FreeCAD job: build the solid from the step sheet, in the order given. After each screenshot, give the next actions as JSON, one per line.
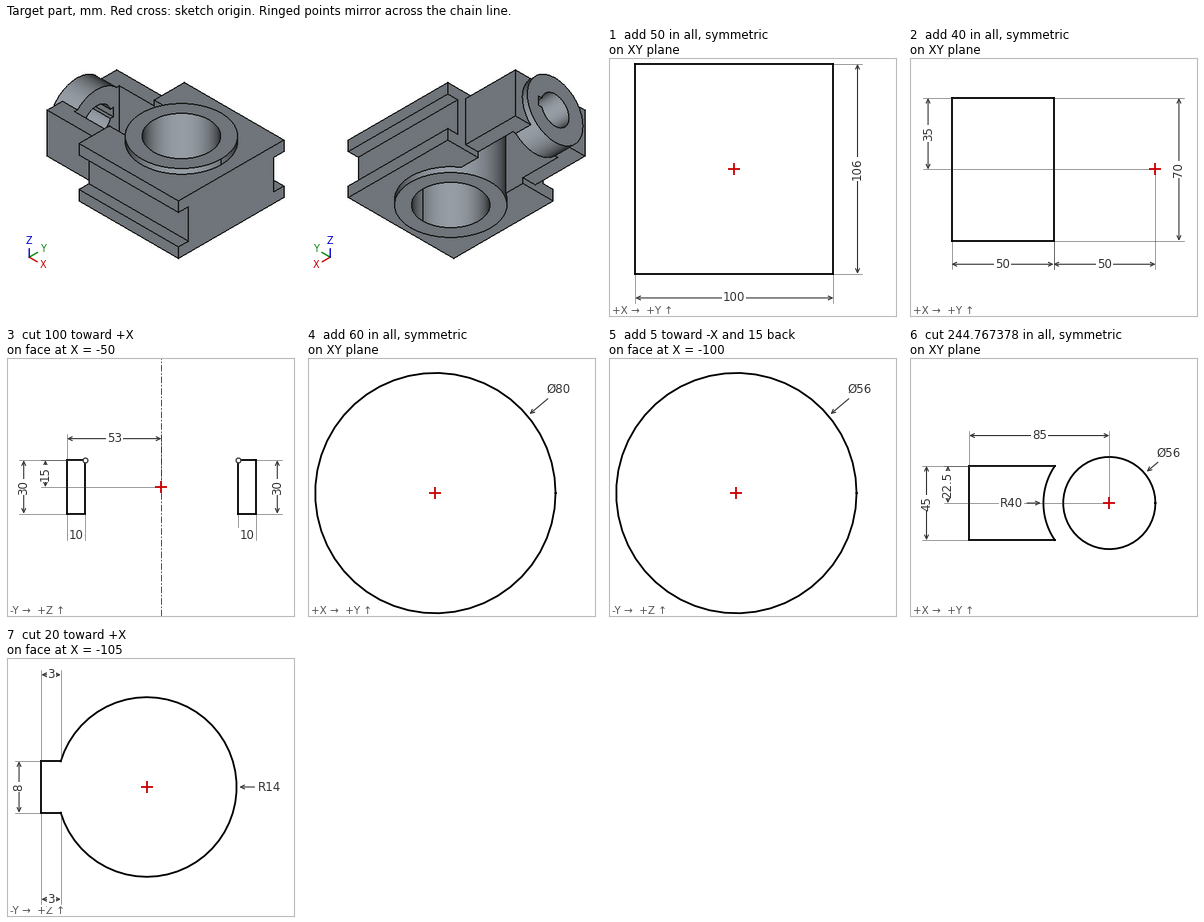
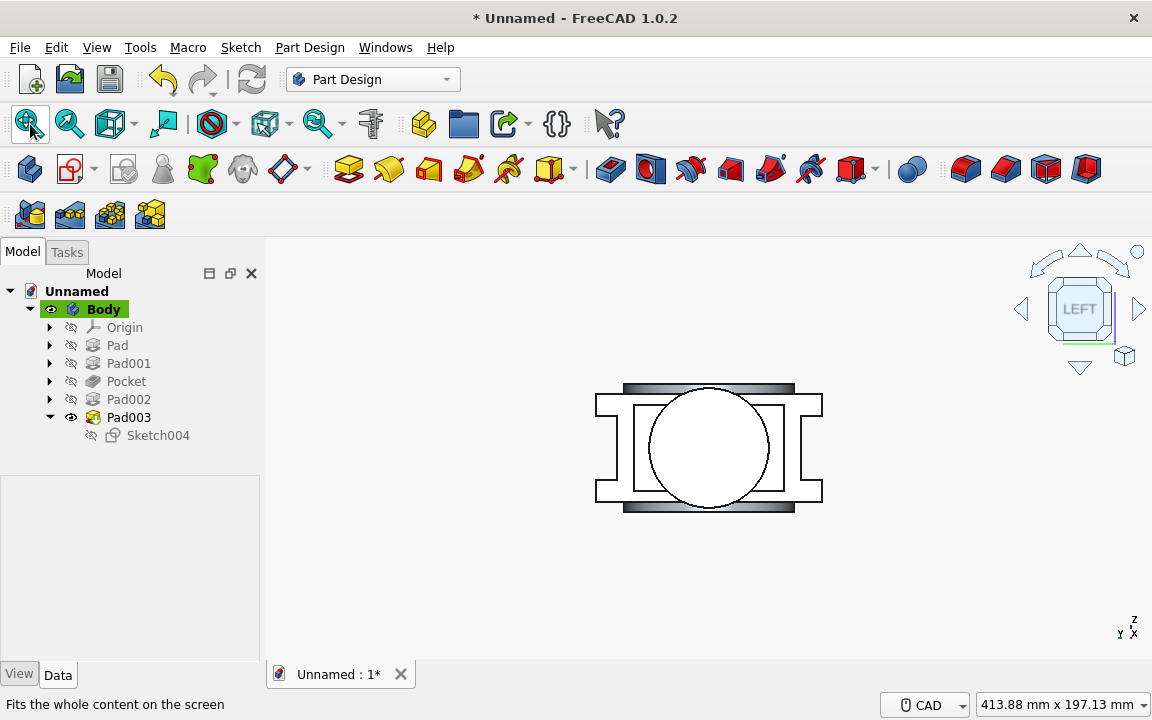
{"action": "left_click", "coordinate": [70, 170]}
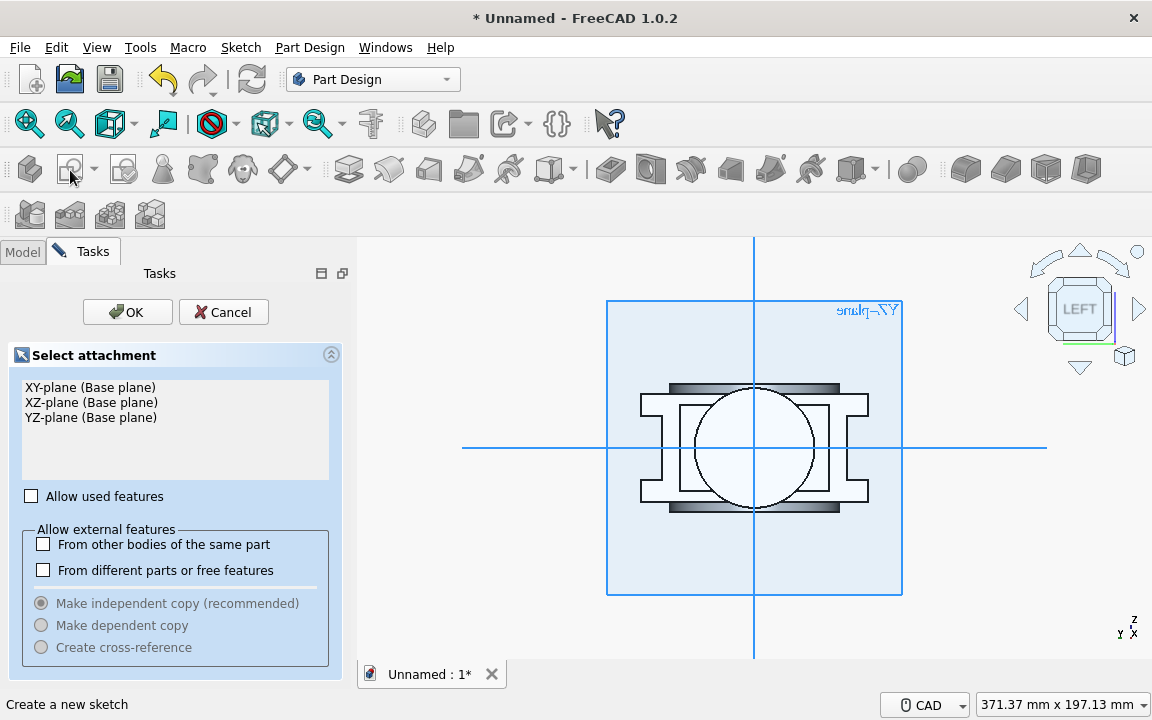
{"action": "left_click", "coordinate": [82, 388]}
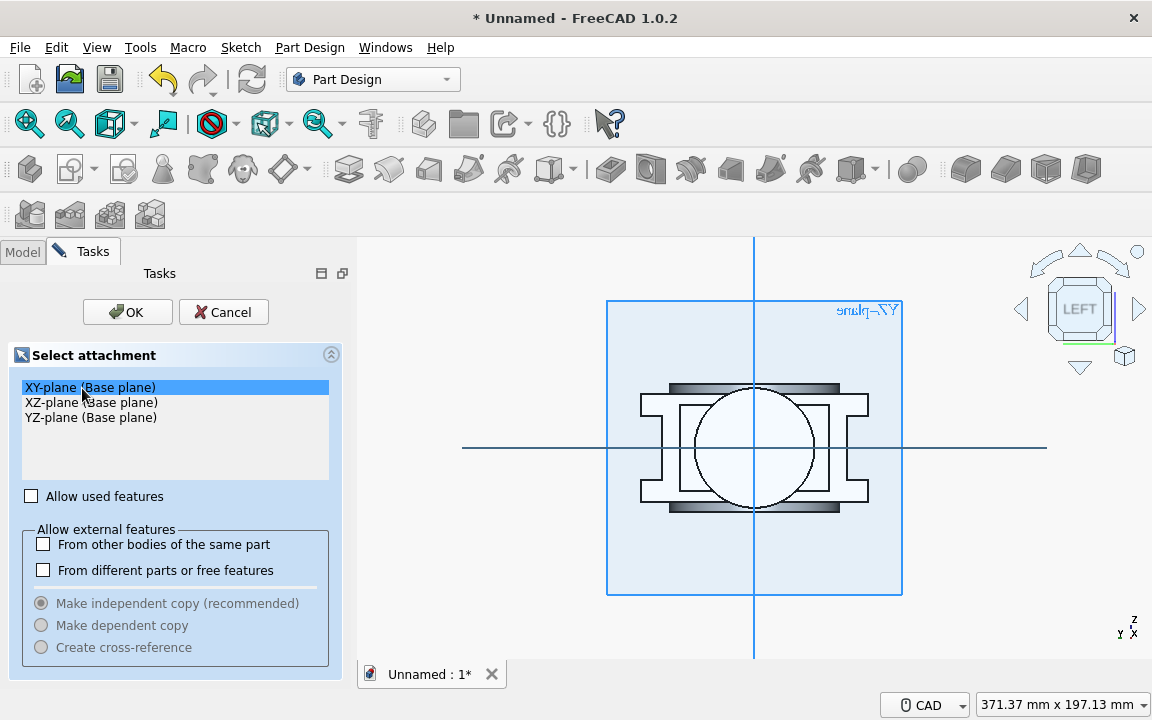
{"action": "left_click", "coordinate": [128, 312]}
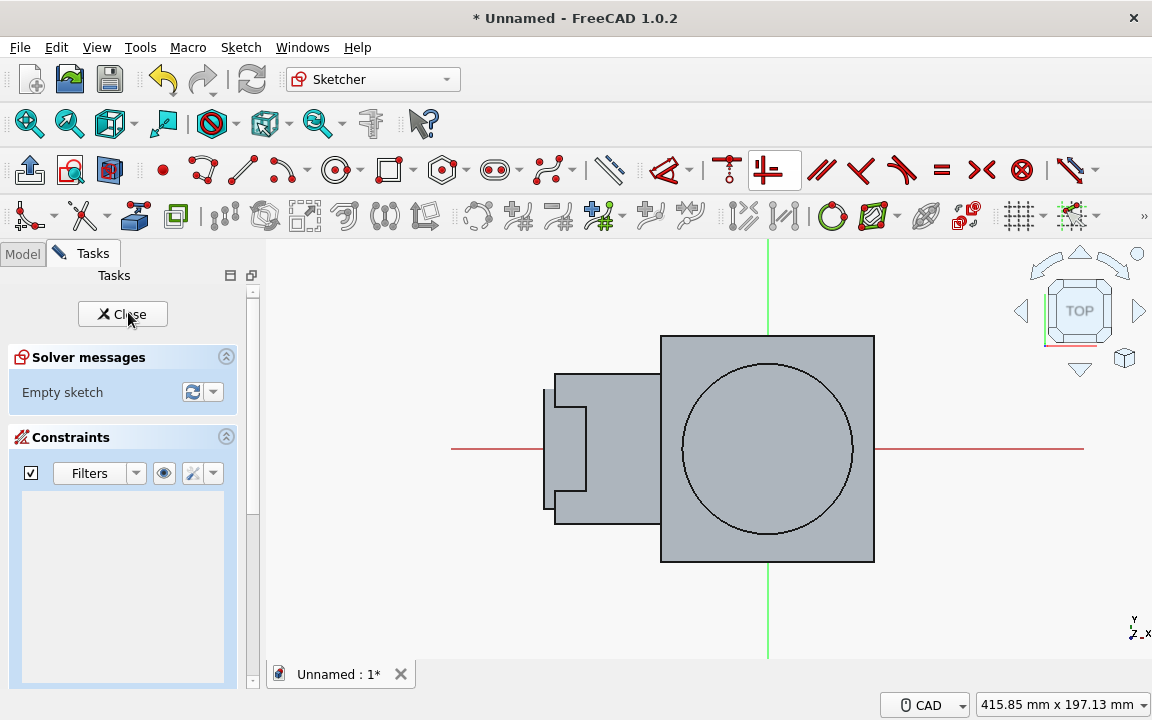
{"action": "left_click", "coordinate": [110, 170]}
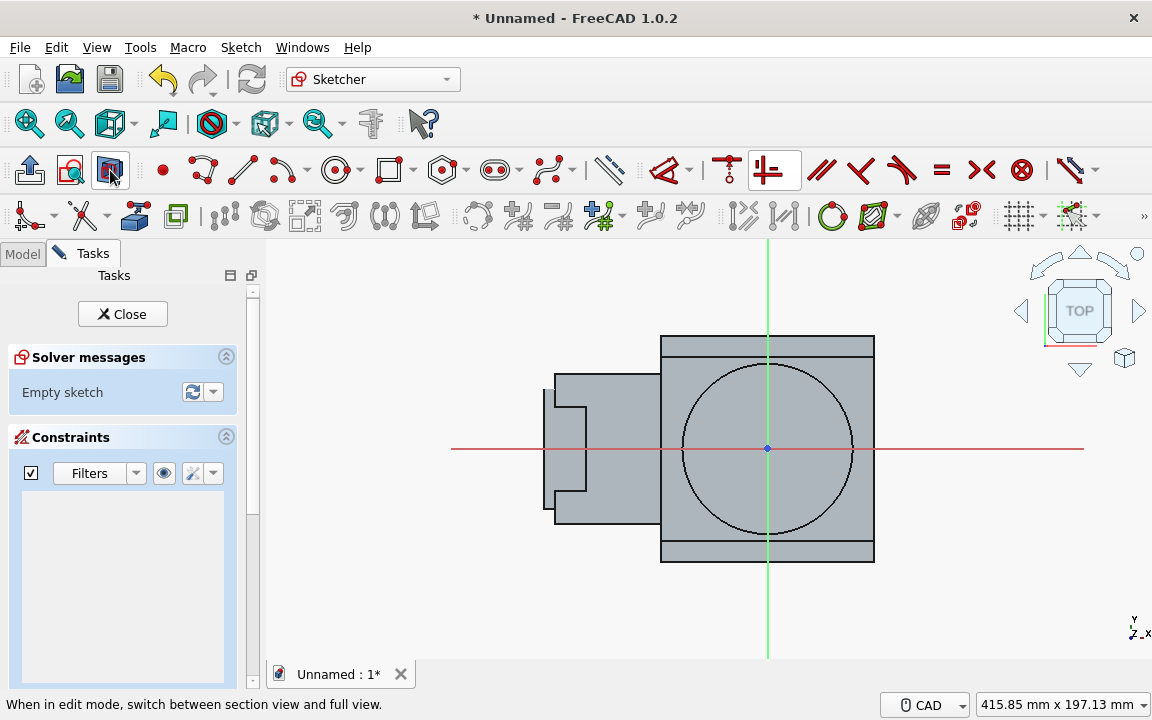
{"action": "scroll", "coordinate": [761, 449], "scroll_direction": "up", "scroll_amount": 4}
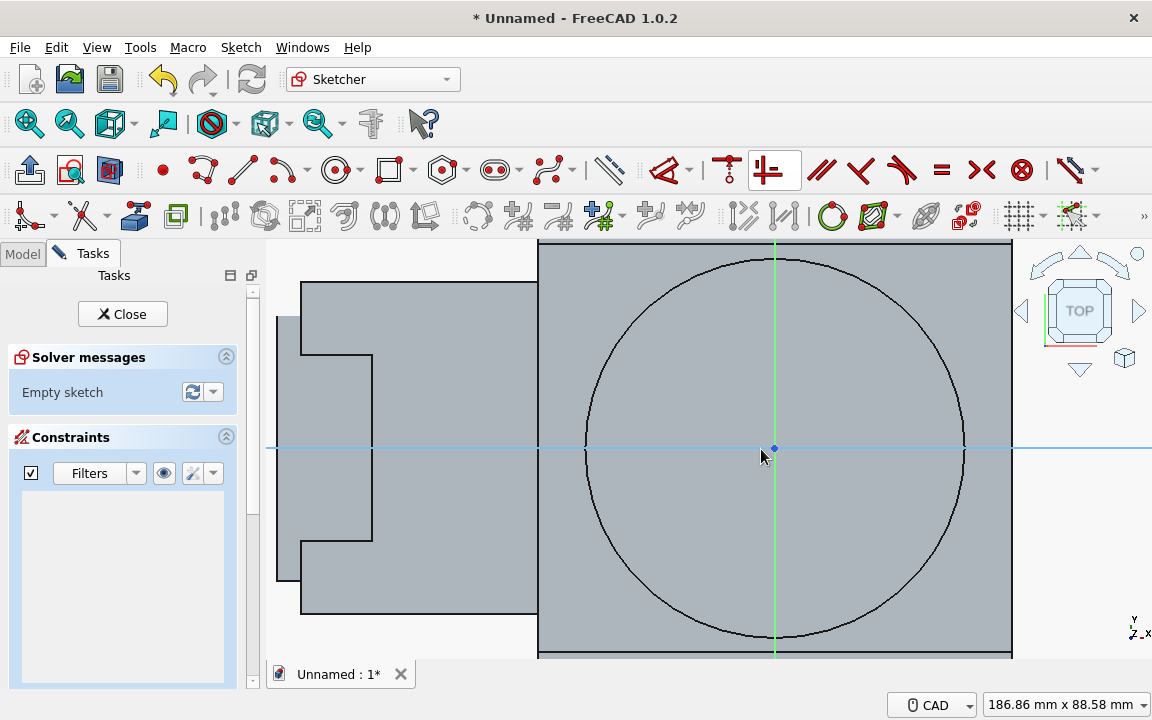
{"action": "left_click", "coordinate": [204, 170]}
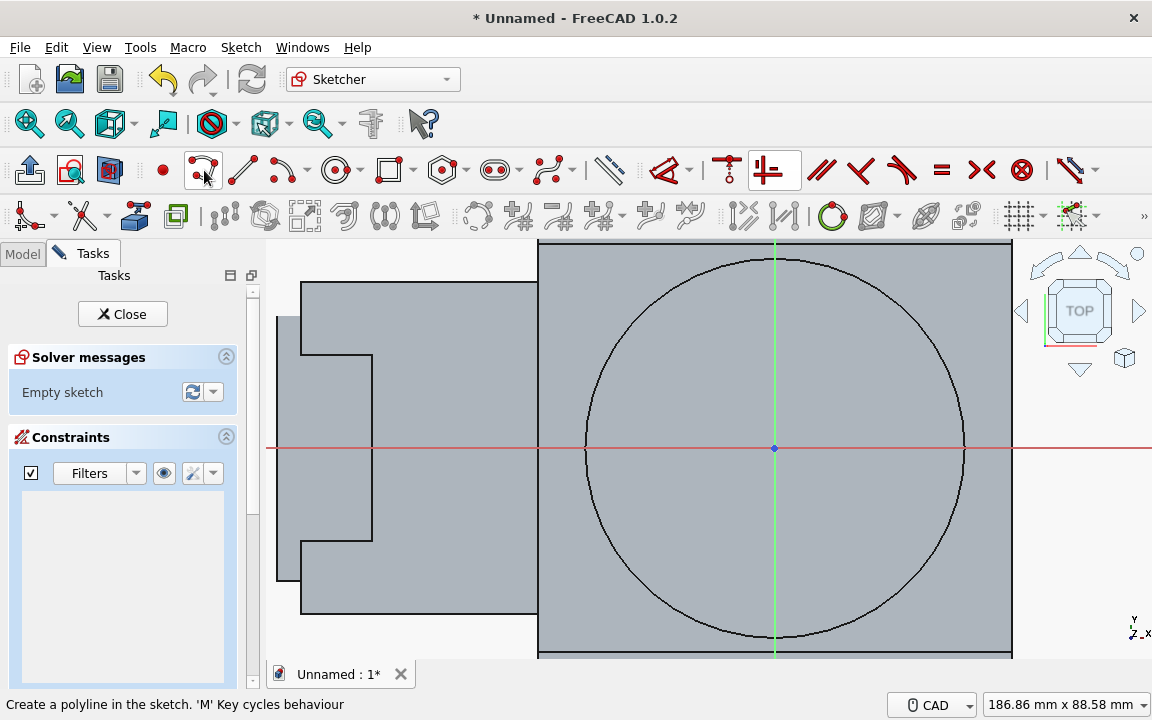
{"action": "left_click", "coordinate": [618, 342]}
{"action": "left_click", "coordinate": [372, 342]}
{"action": "left_click", "coordinate": [372, 555]}
{"action": "left_click", "coordinate": [618, 555]}
{"action": "right_click", "coordinate": [618, 555]}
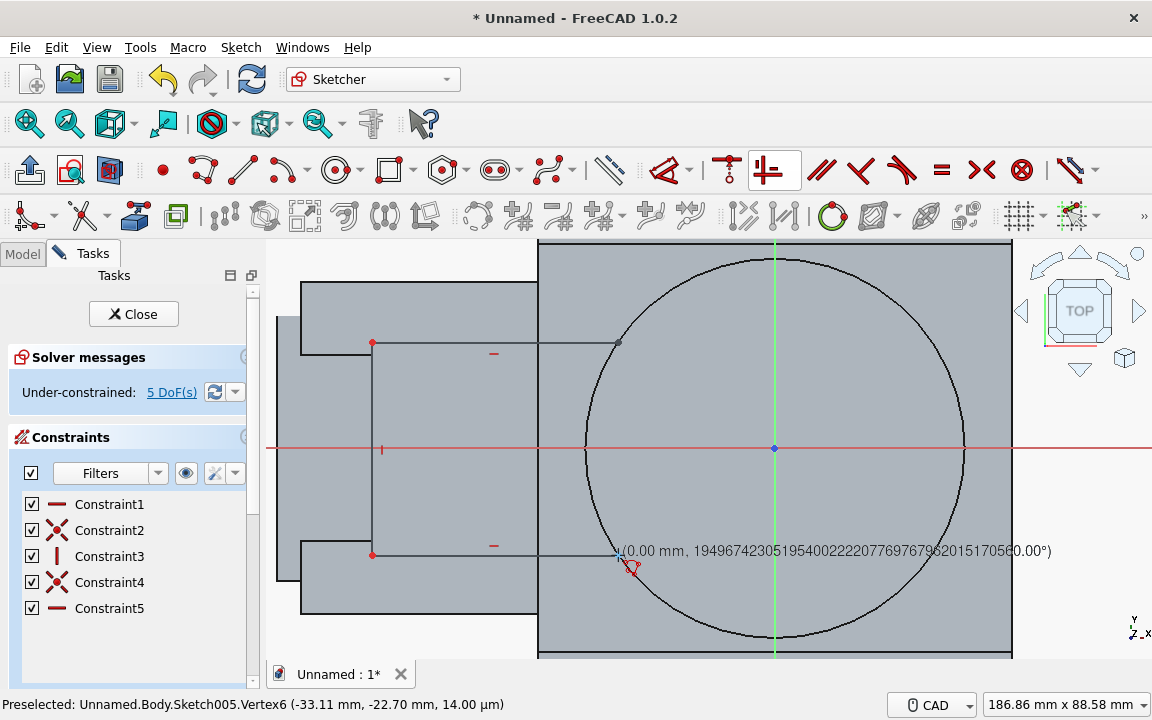
{"action": "key", "text": "g 3 a"}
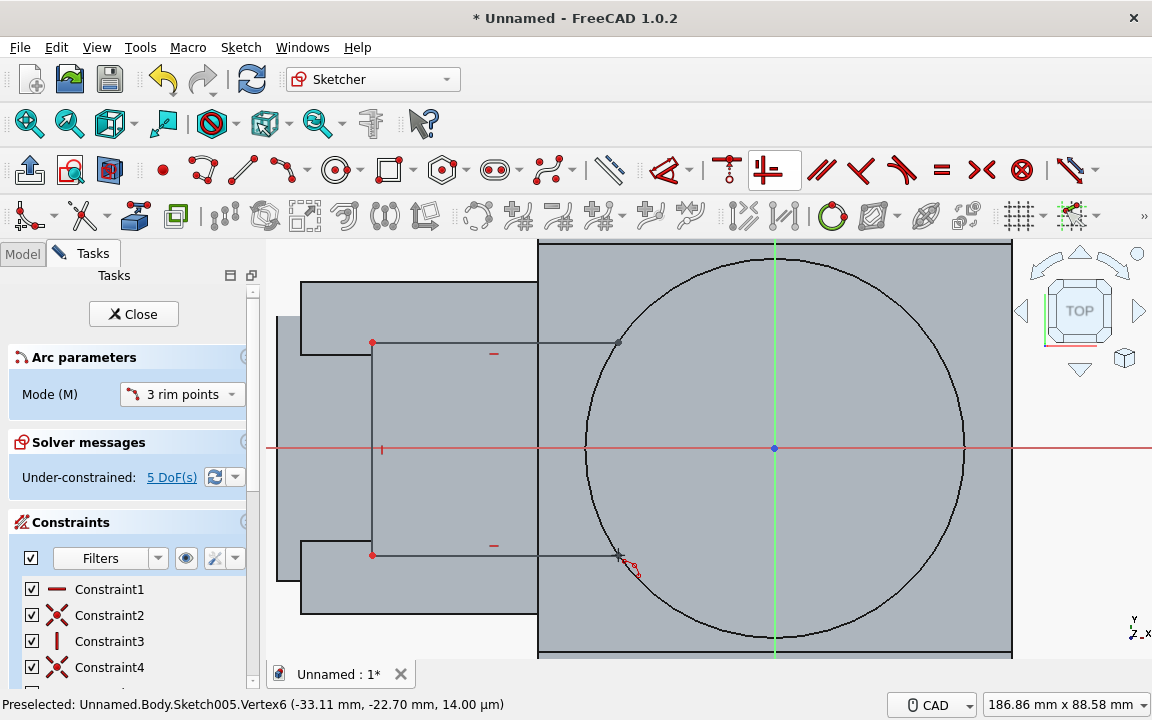
{"action": "left_click", "coordinate": [618, 556]}
{"action": "left_click", "coordinate": [618, 343]}
{"action": "left_click", "coordinate": [587, 426]}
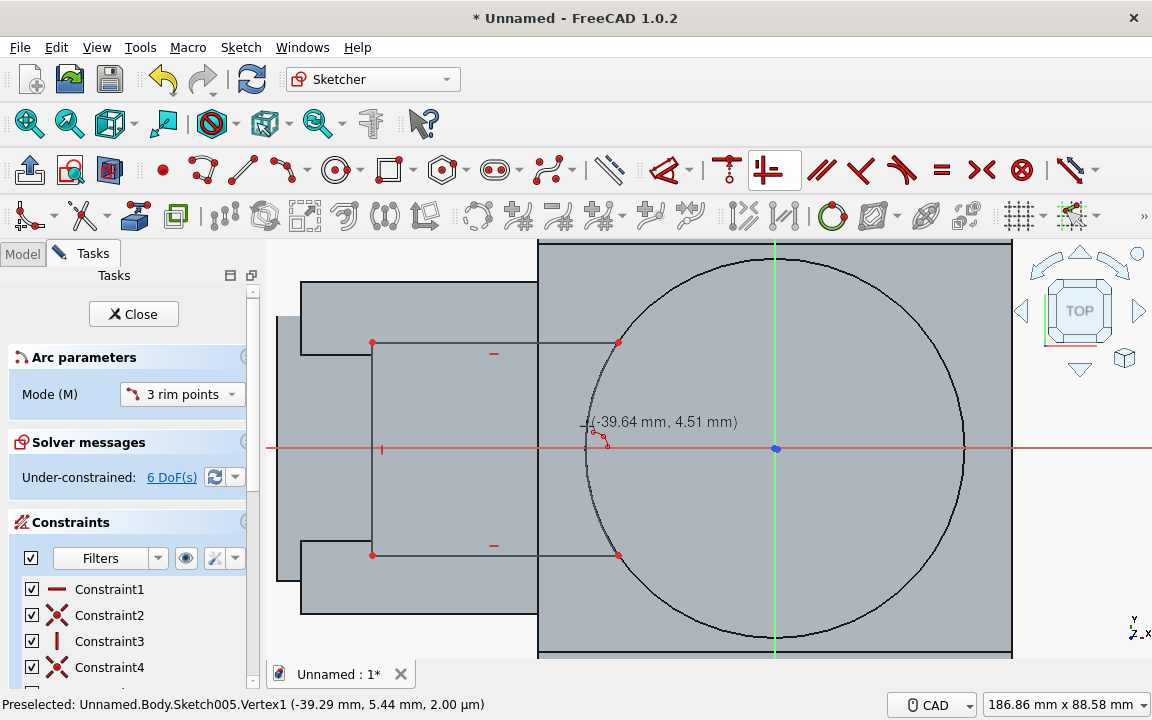
{"action": "left_click", "coordinate": [336, 170]}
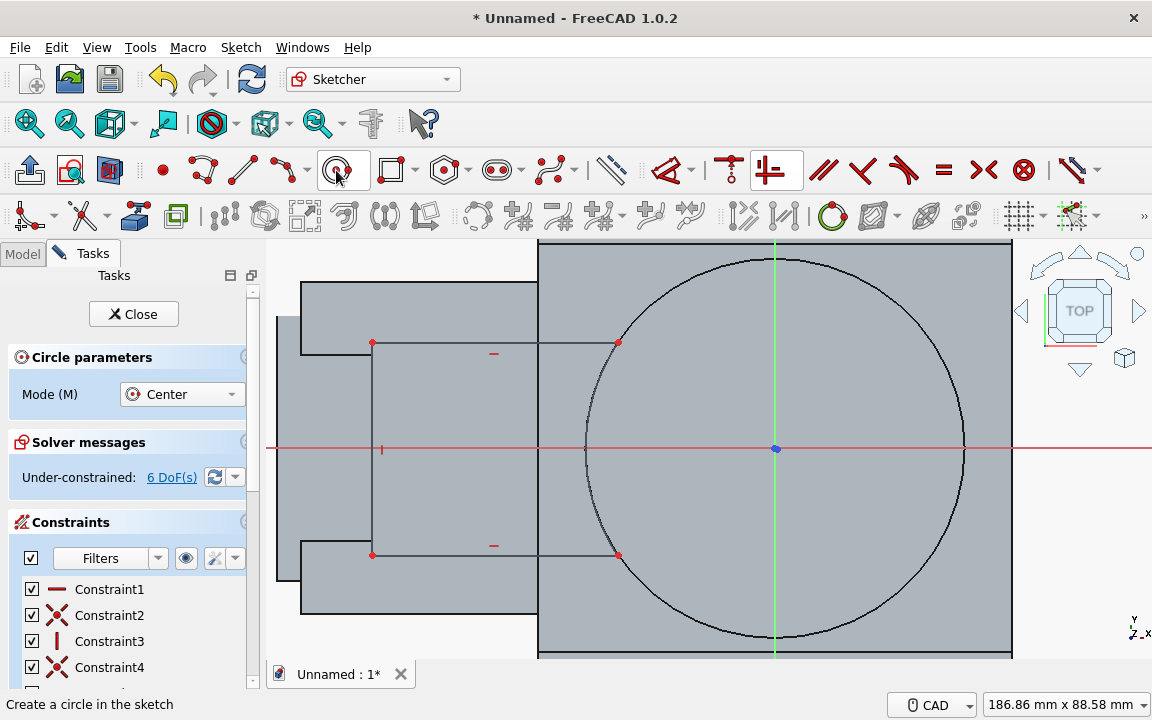
{"action": "left_click", "coordinate": [775, 448]}
{"action": "mouse_move", "coordinate": [869, 355]}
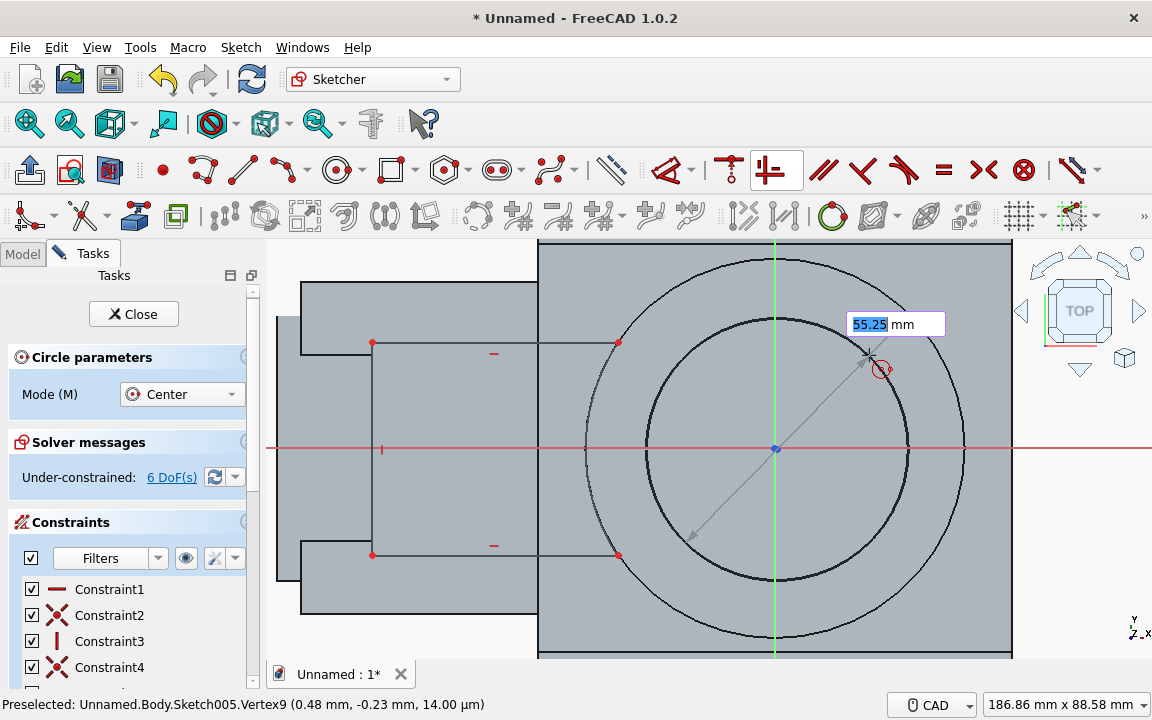
{"action": "type", "text": "56"}
{"action": "key", "text": "Return"}
{"action": "key", "text": "Escape"}